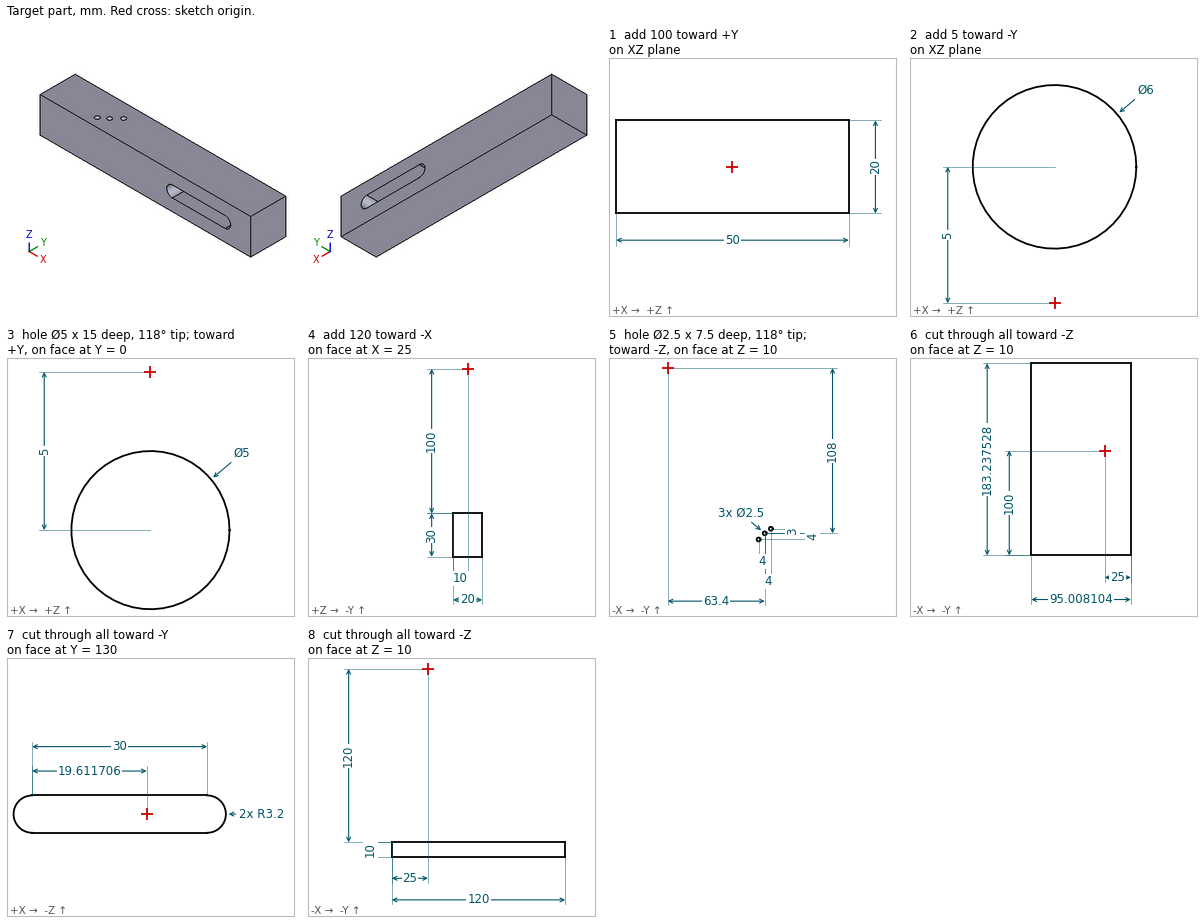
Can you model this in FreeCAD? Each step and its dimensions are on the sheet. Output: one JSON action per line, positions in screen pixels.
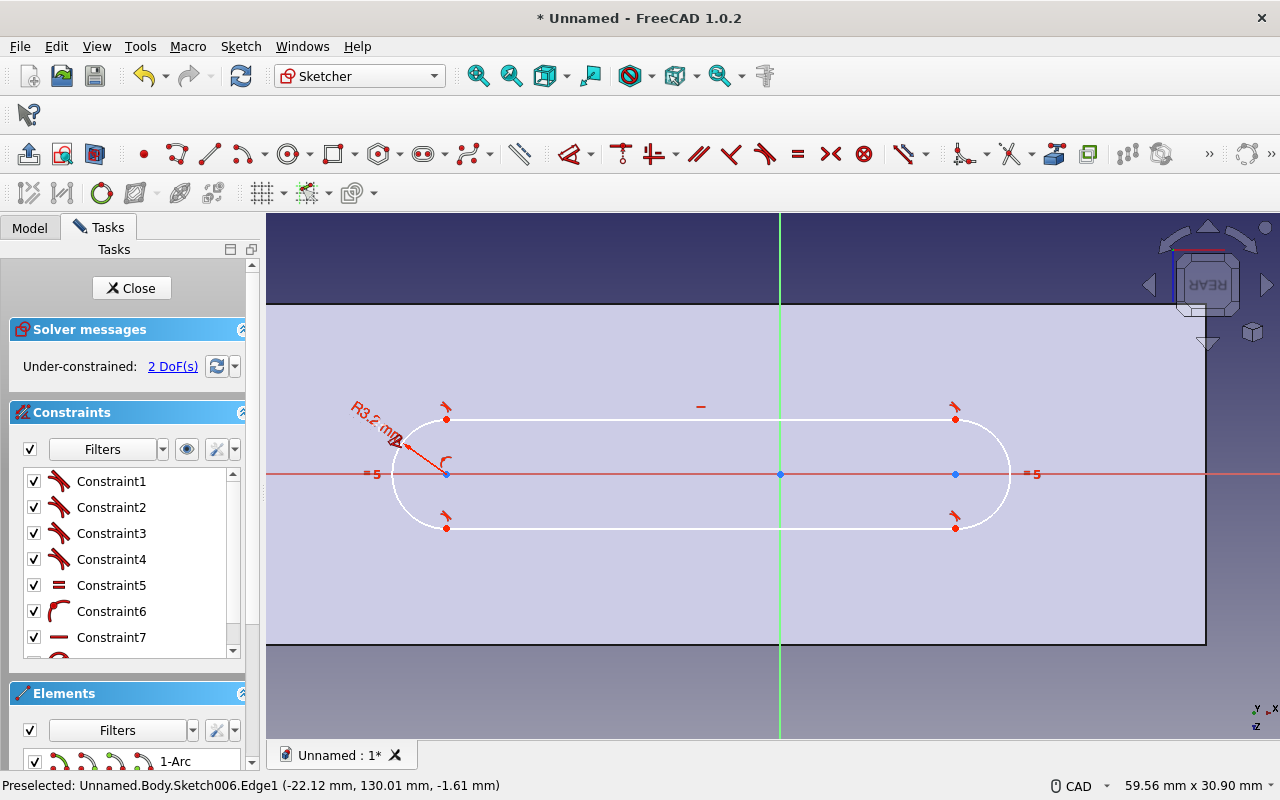
{"action": "left_click", "coordinate": [600, 420]}
{"action": "left_click", "coordinate": [701, 386]}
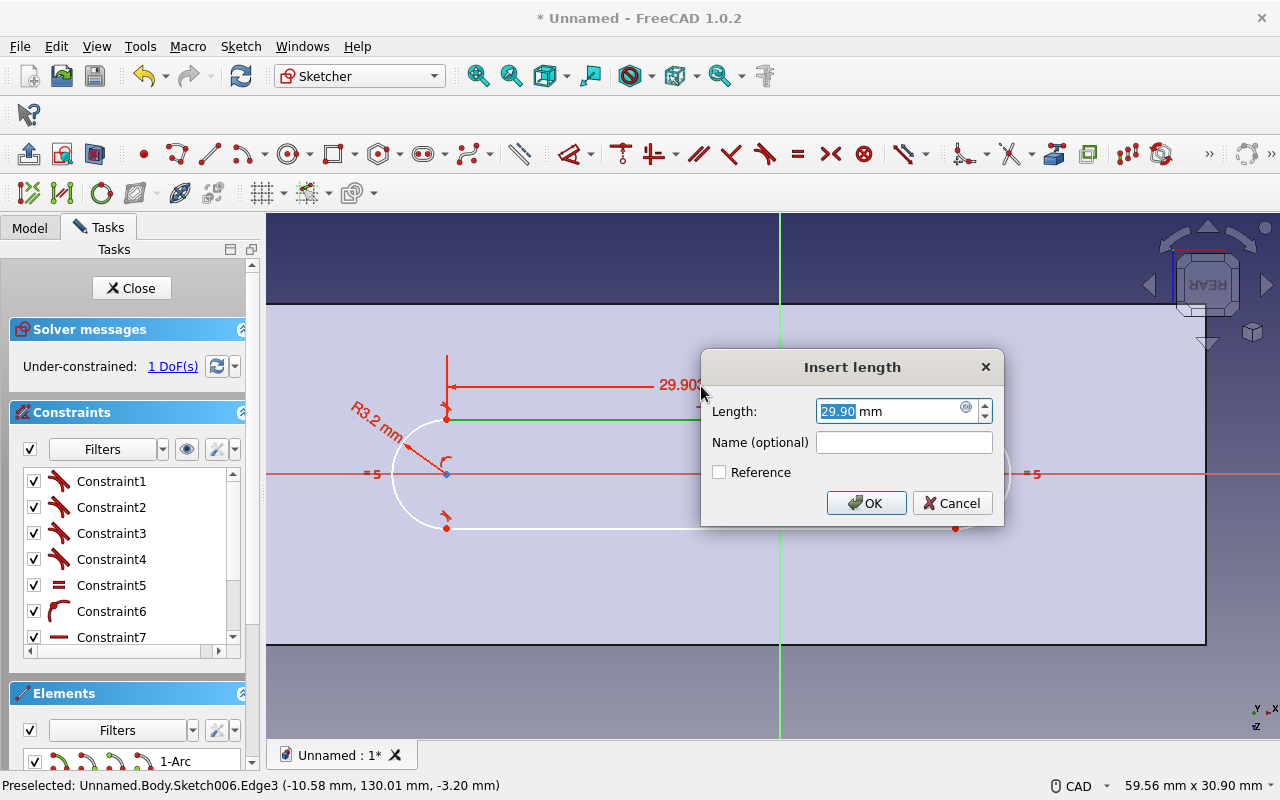
{"action": "type", "text": "30"}
{"action": "key", "text": "Return"}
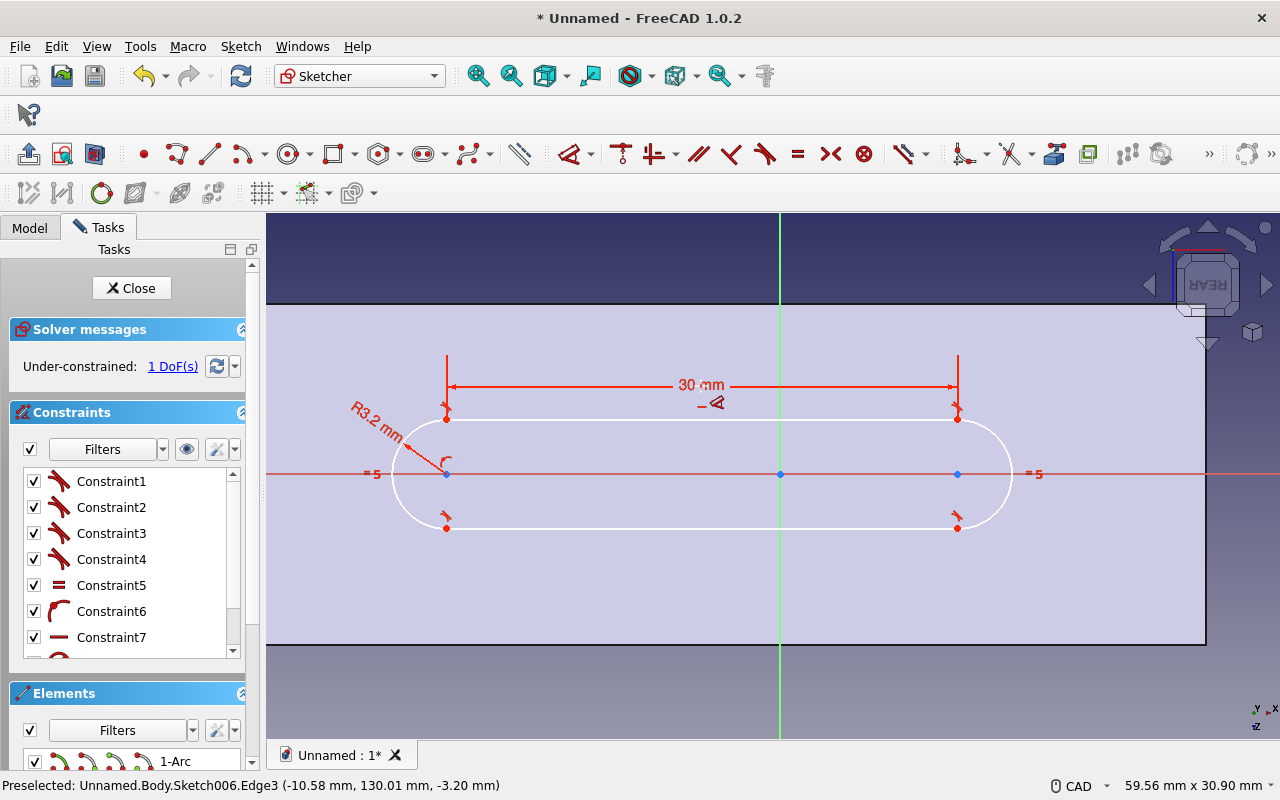
{"action": "left_click", "coordinate": [447, 420]}
{"action": "left_click", "coordinate": [613, 386]}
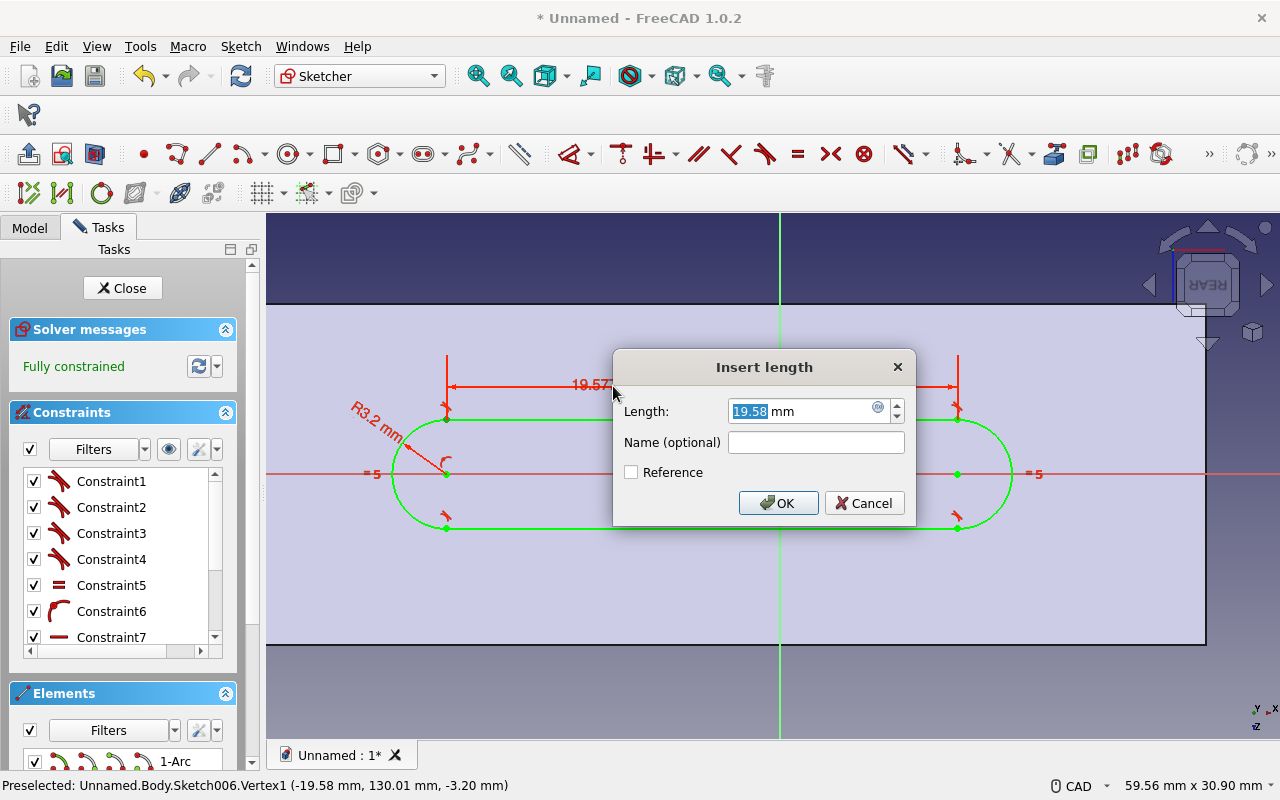
{"action": "type", "text": "19.611706"}
{"action": "key", "text": "Return"}
{"action": "key", "text": "Escape"}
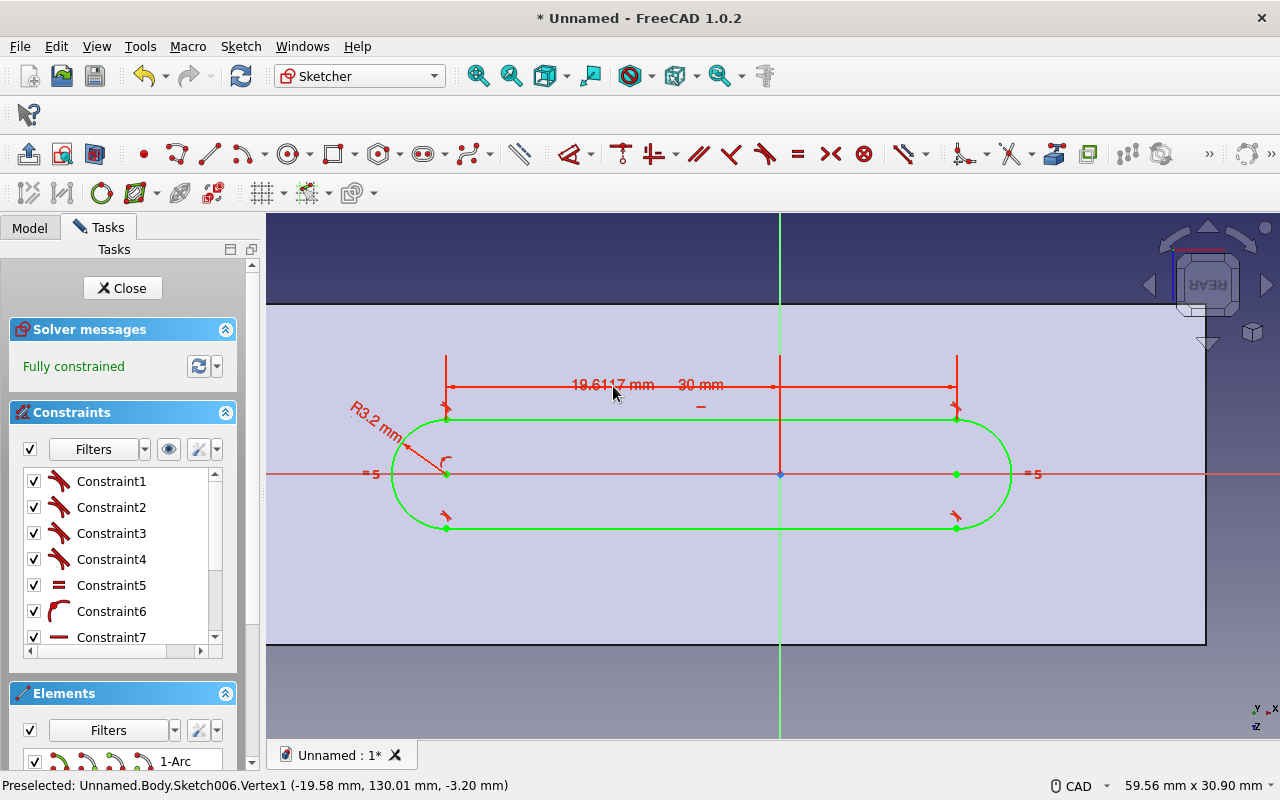
{"action": "left_click", "coordinate": [123, 288]}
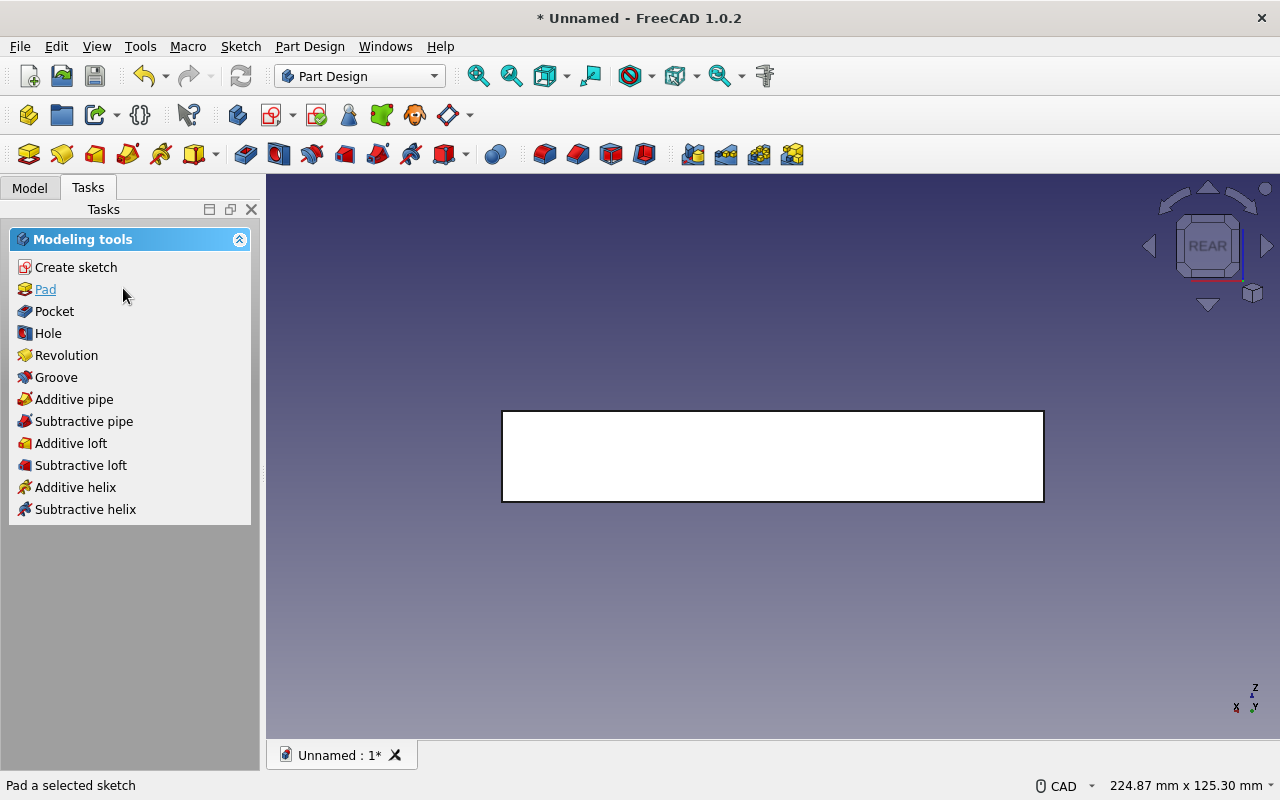
{"action": "left_click", "coordinate": [246, 154]}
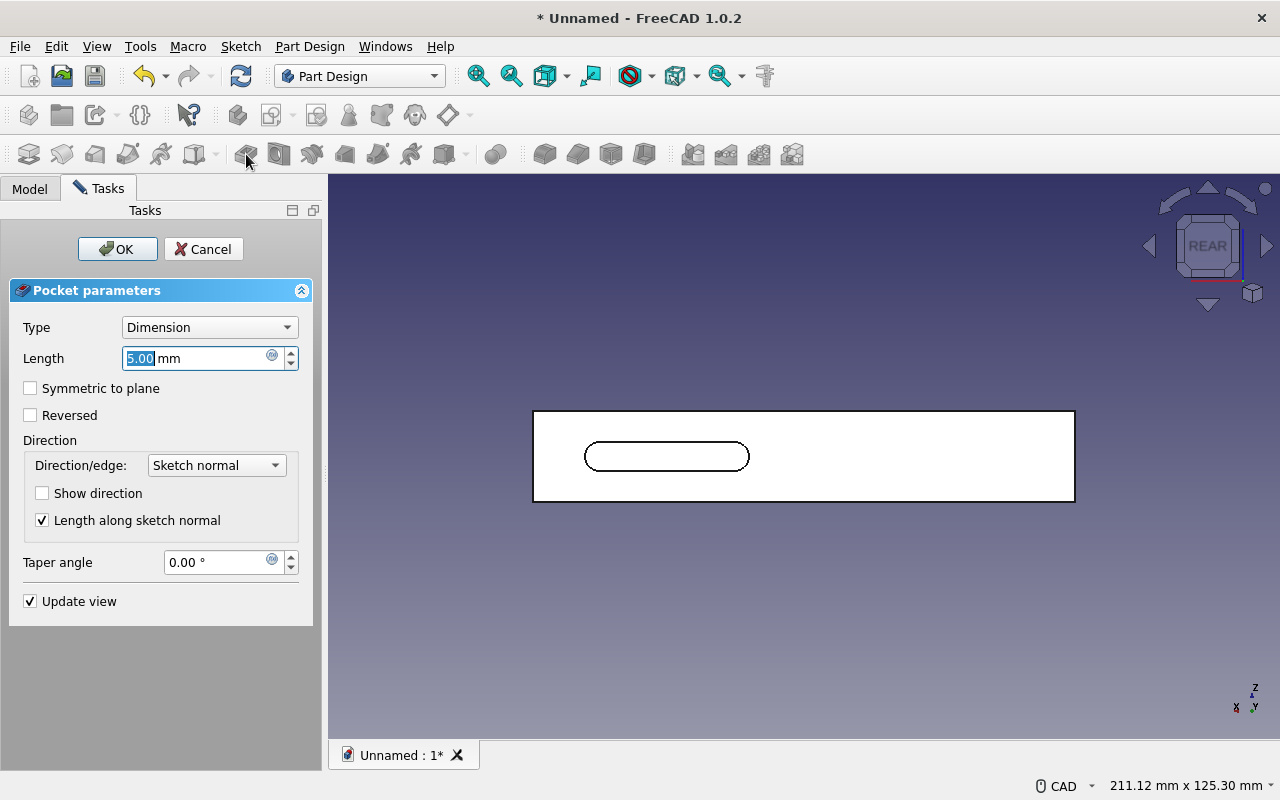
{"action": "left_click", "coordinate": [210, 328]}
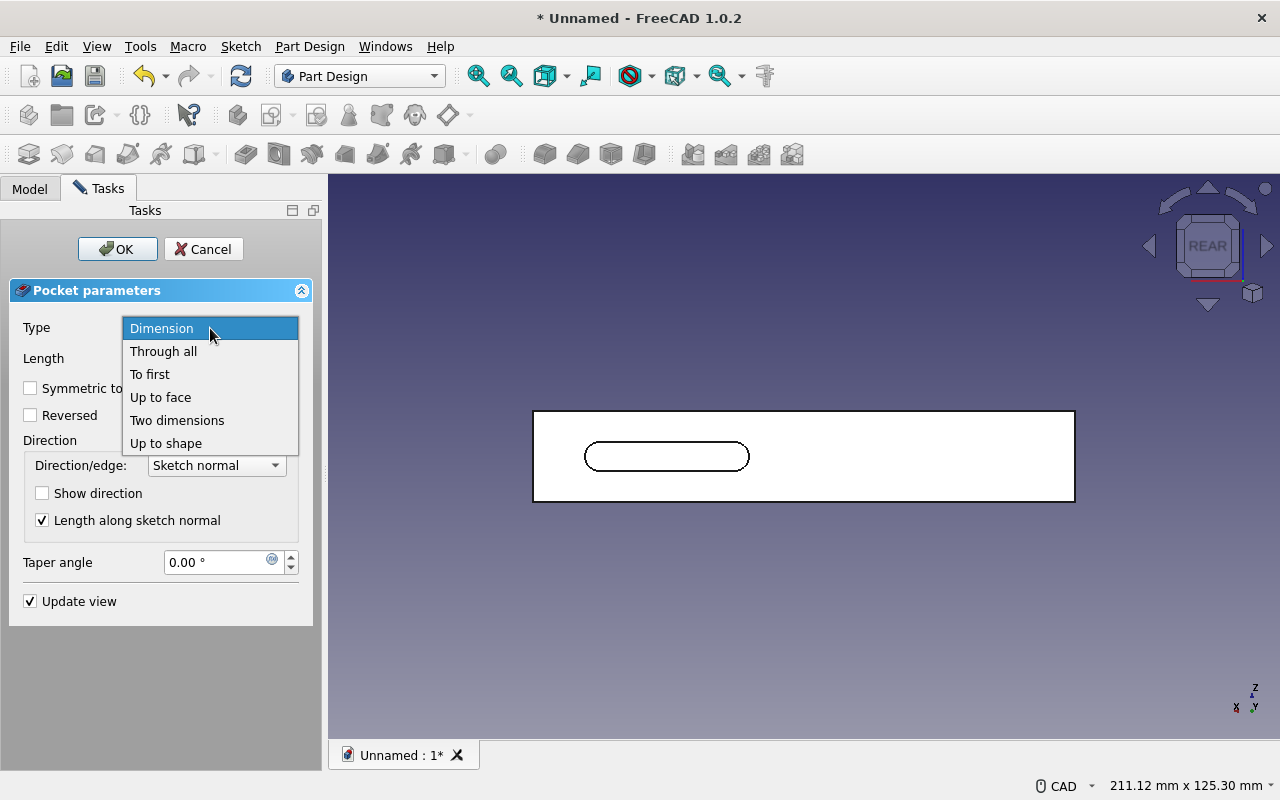
{"action": "left_click", "coordinate": [208, 352]}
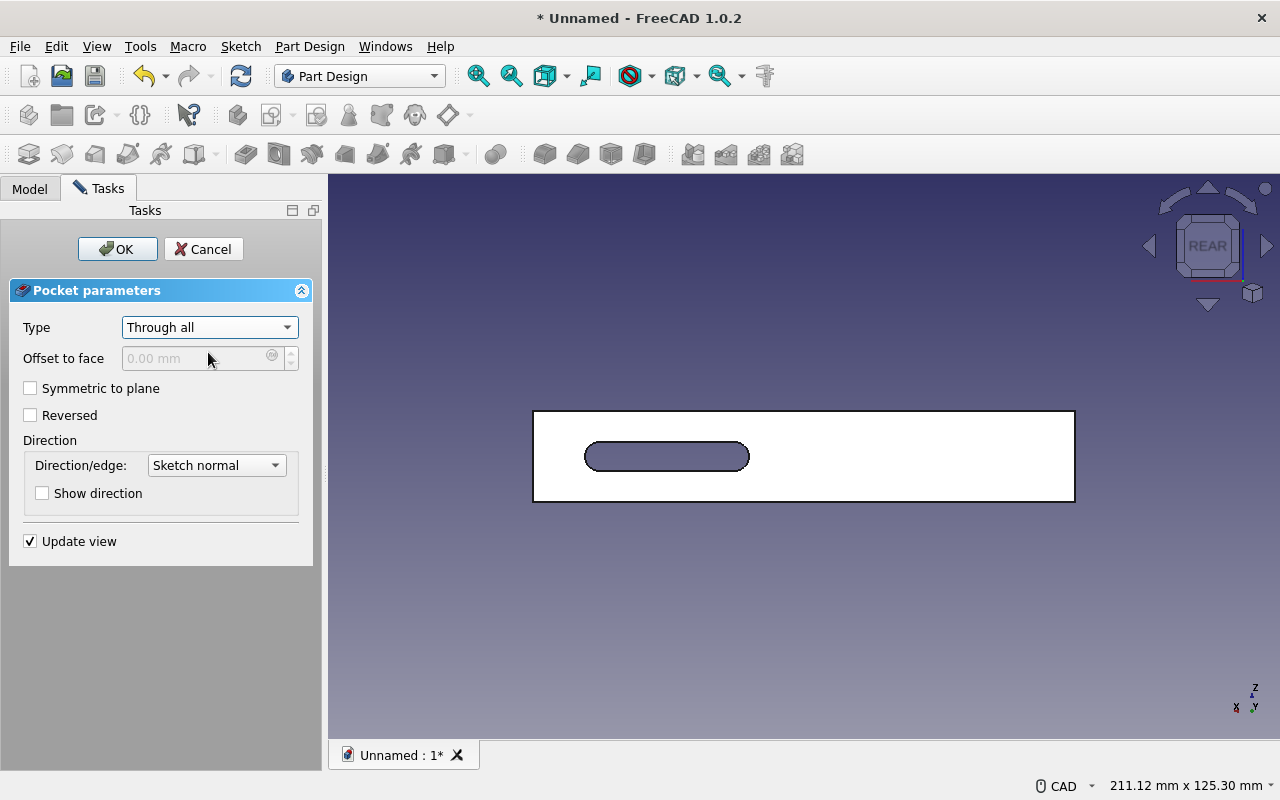
{"action": "left_click", "coordinate": [118, 249]}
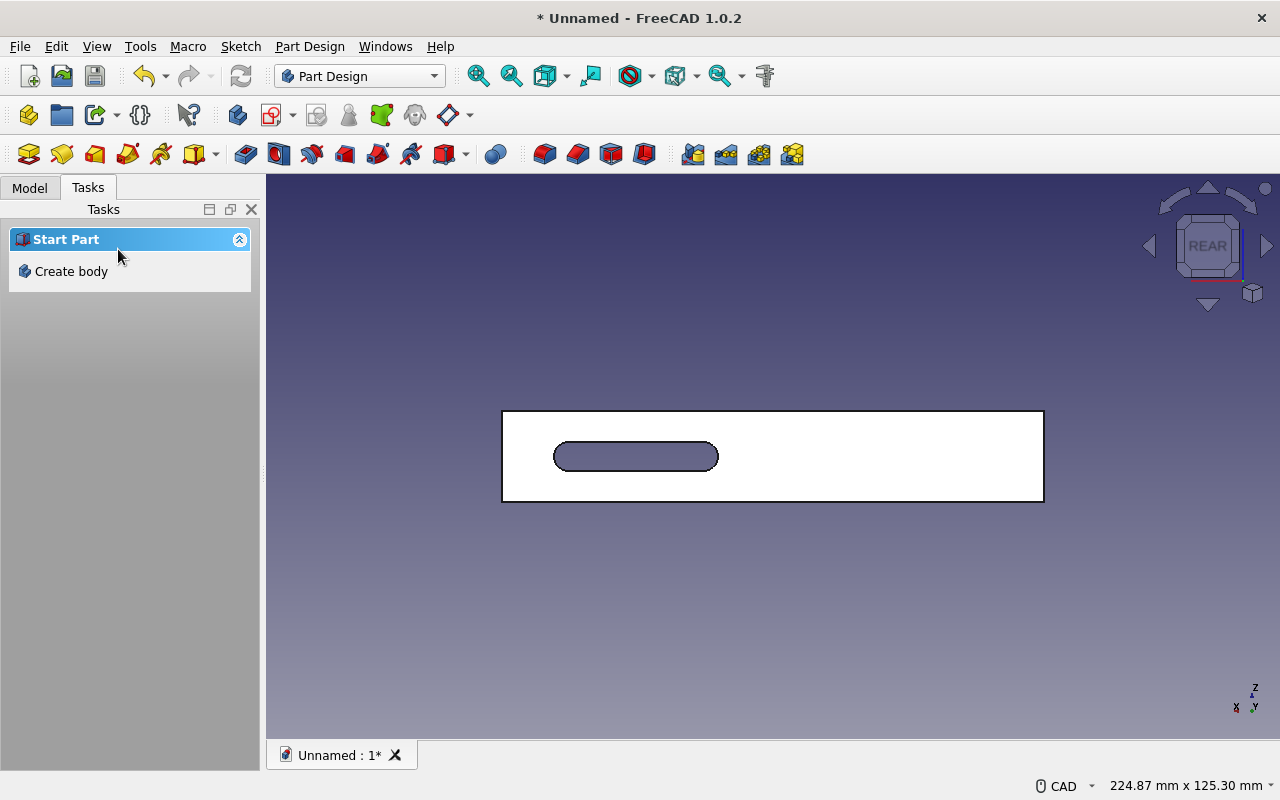
{"action": "key", "text": "0"}